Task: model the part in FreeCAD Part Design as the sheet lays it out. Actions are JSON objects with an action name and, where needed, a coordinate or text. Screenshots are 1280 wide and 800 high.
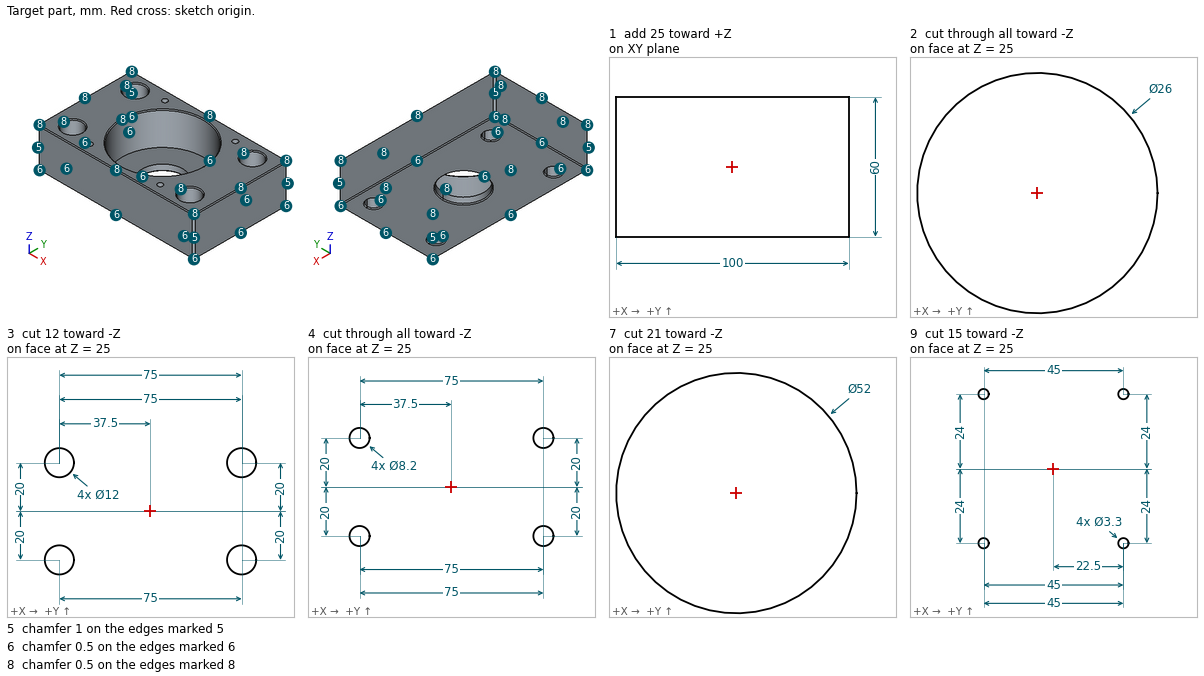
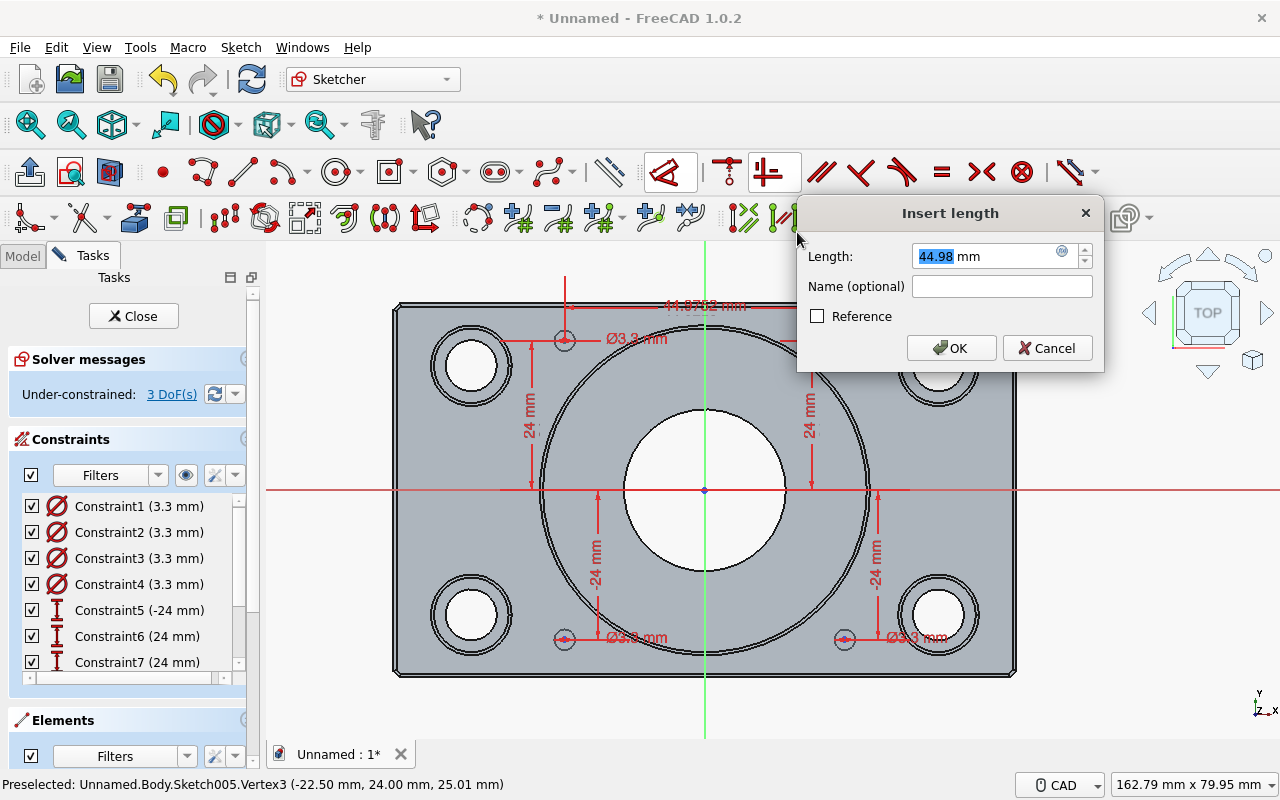
{"action": "type", "text": "45"}
{"action": "key", "text": "Return"}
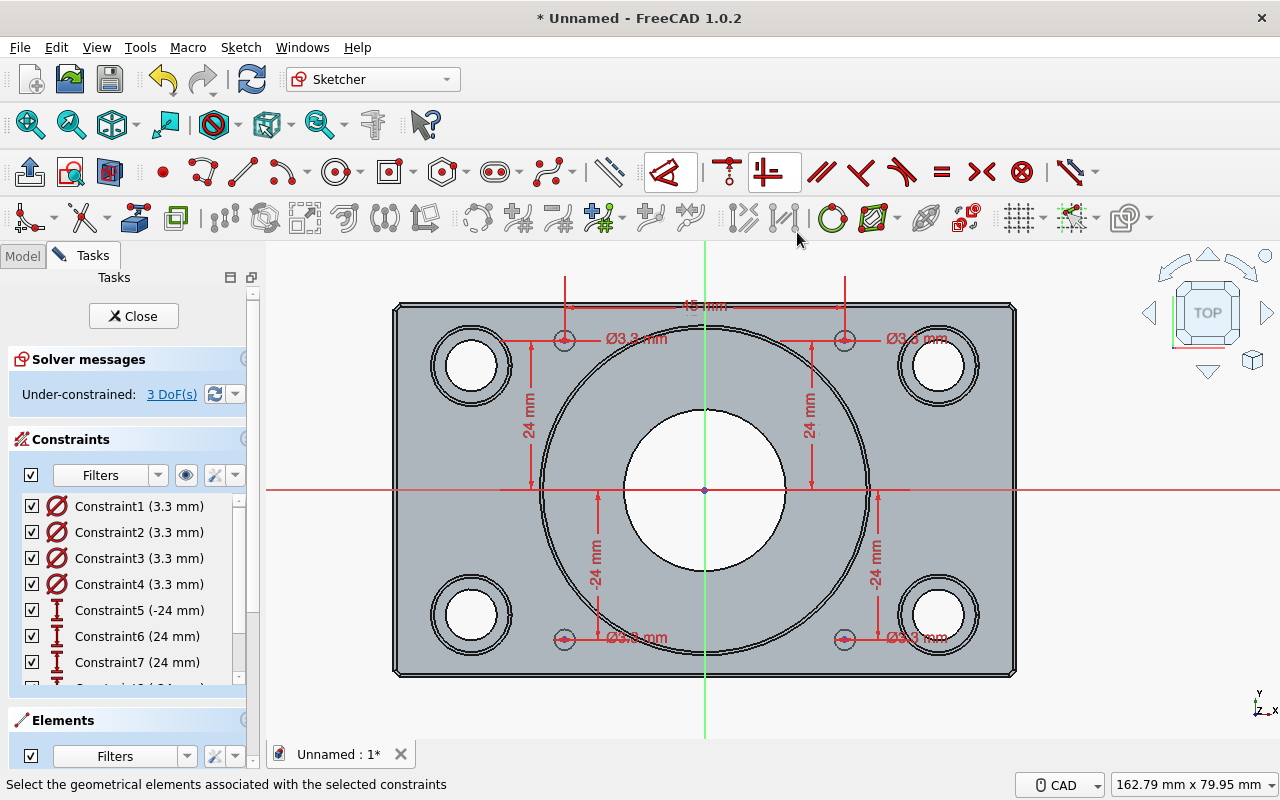
{"action": "left_click", "coordinate": [845, 640]}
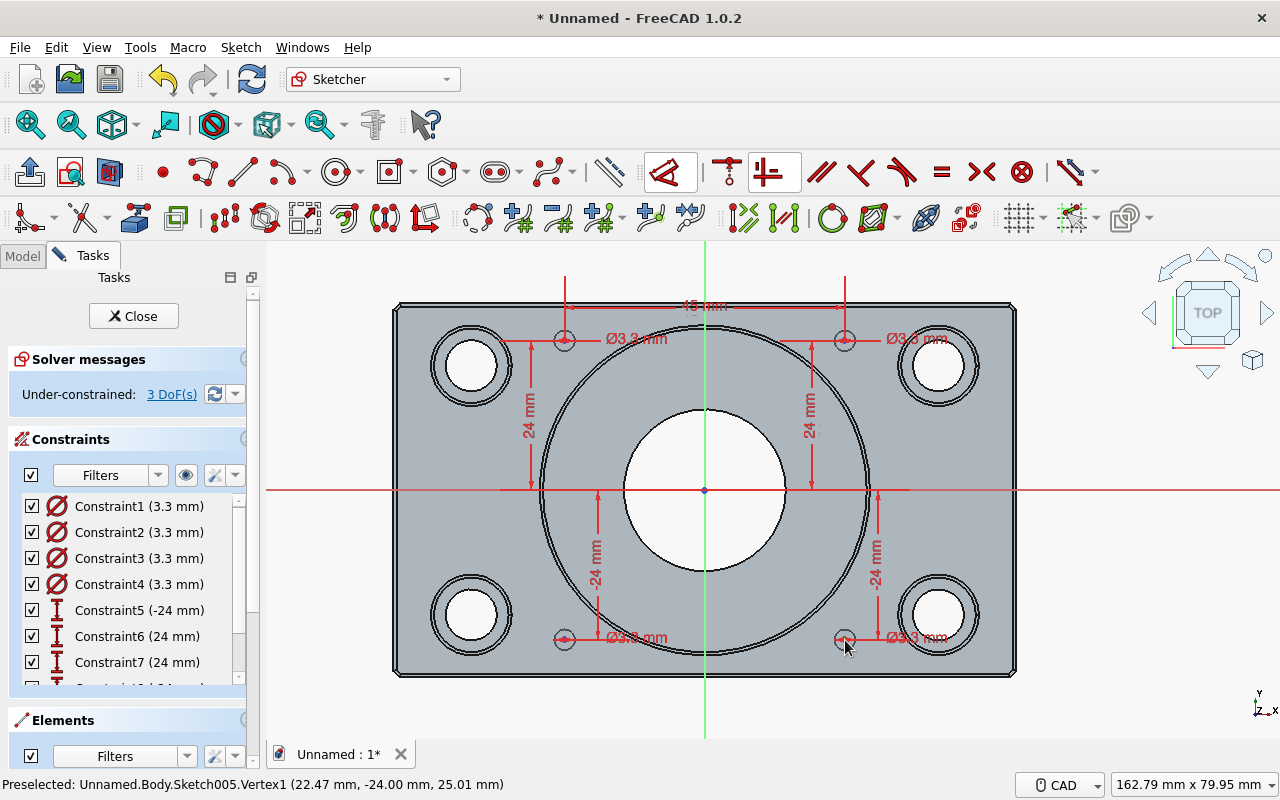
{"action": "left_click", "coordinate": [565, 341]}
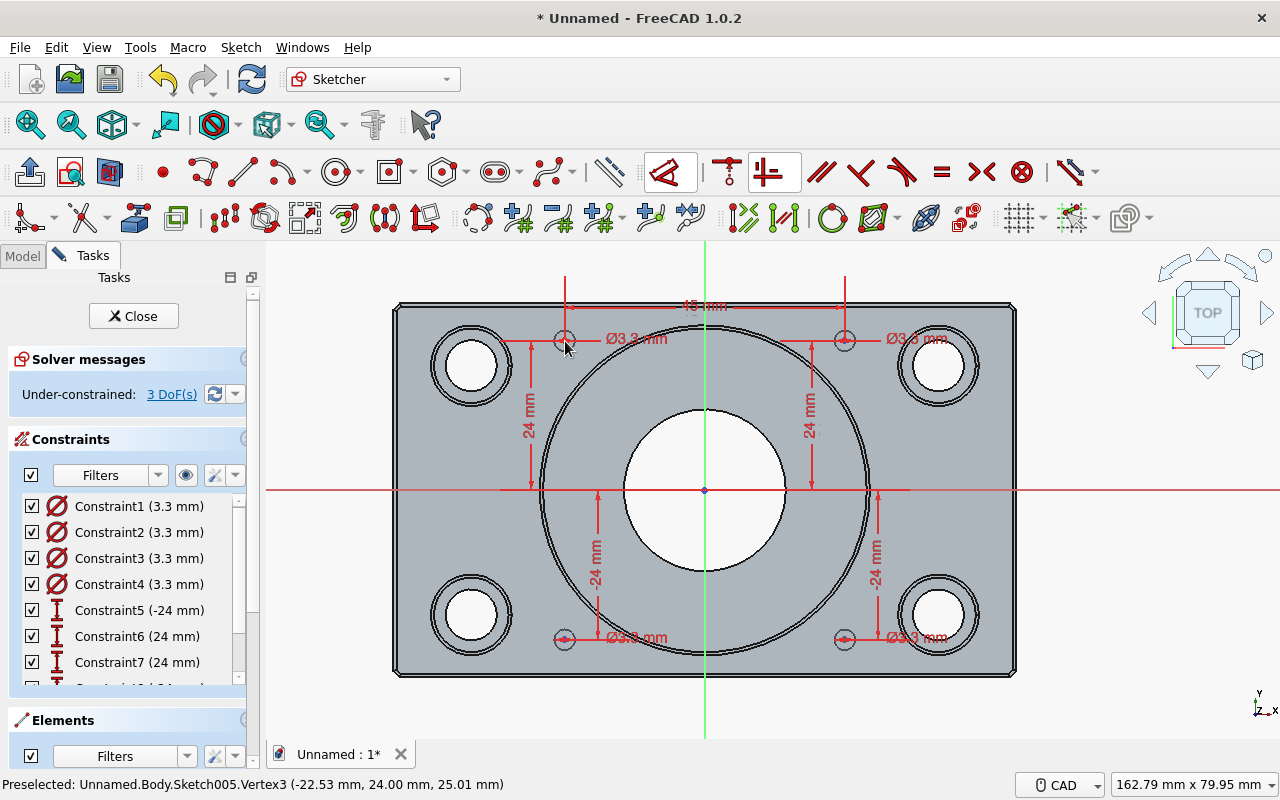
{"action": "left_click", "coordinate": [692, 172]}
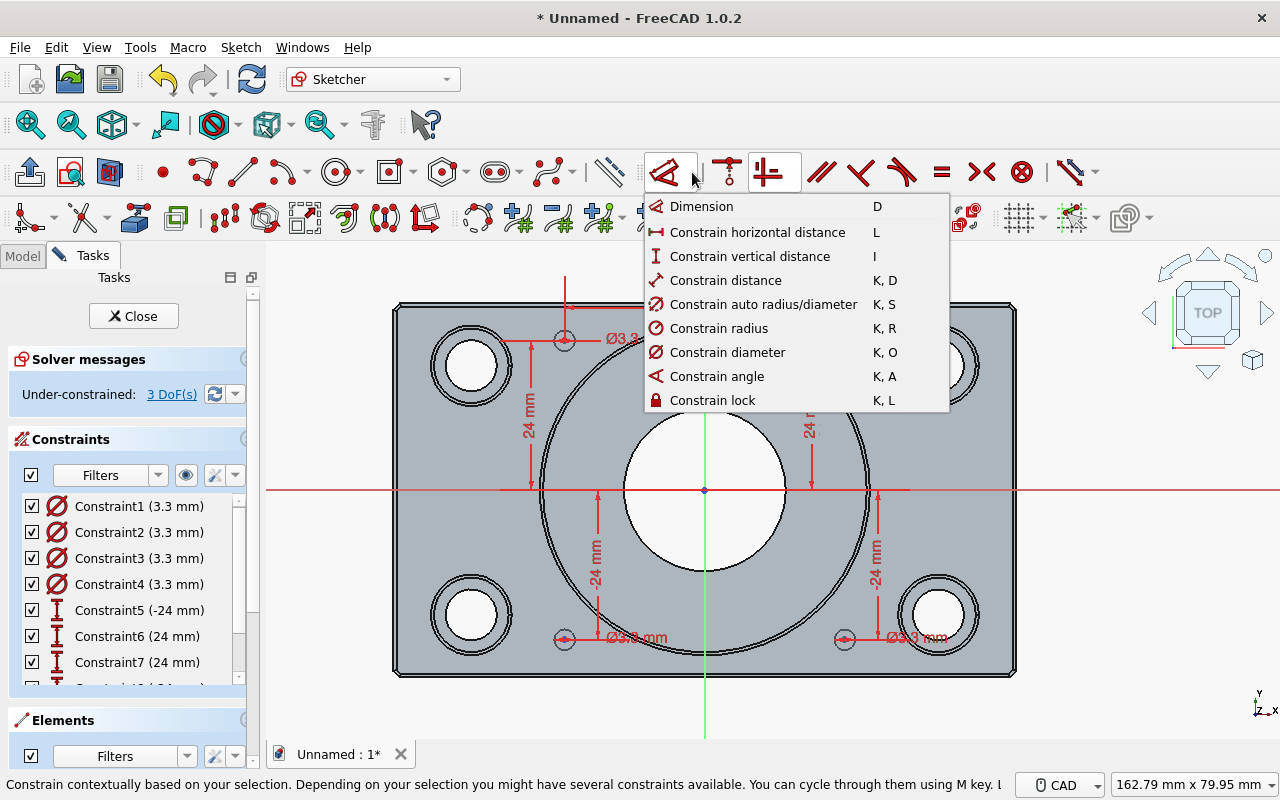
{"action": "left_click", "coordinate": [797, 232]}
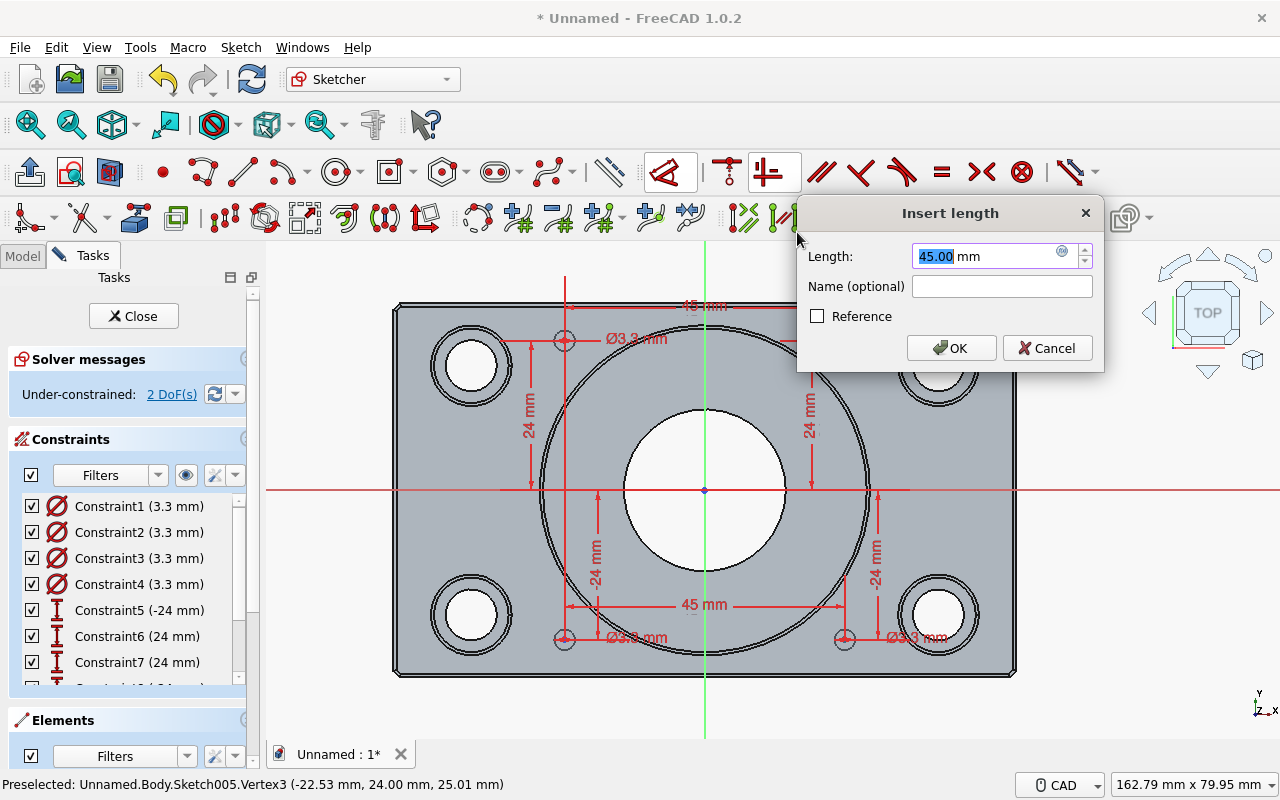
{"action": "type", "text": "45"}
{"action": "key", "text": "Return"}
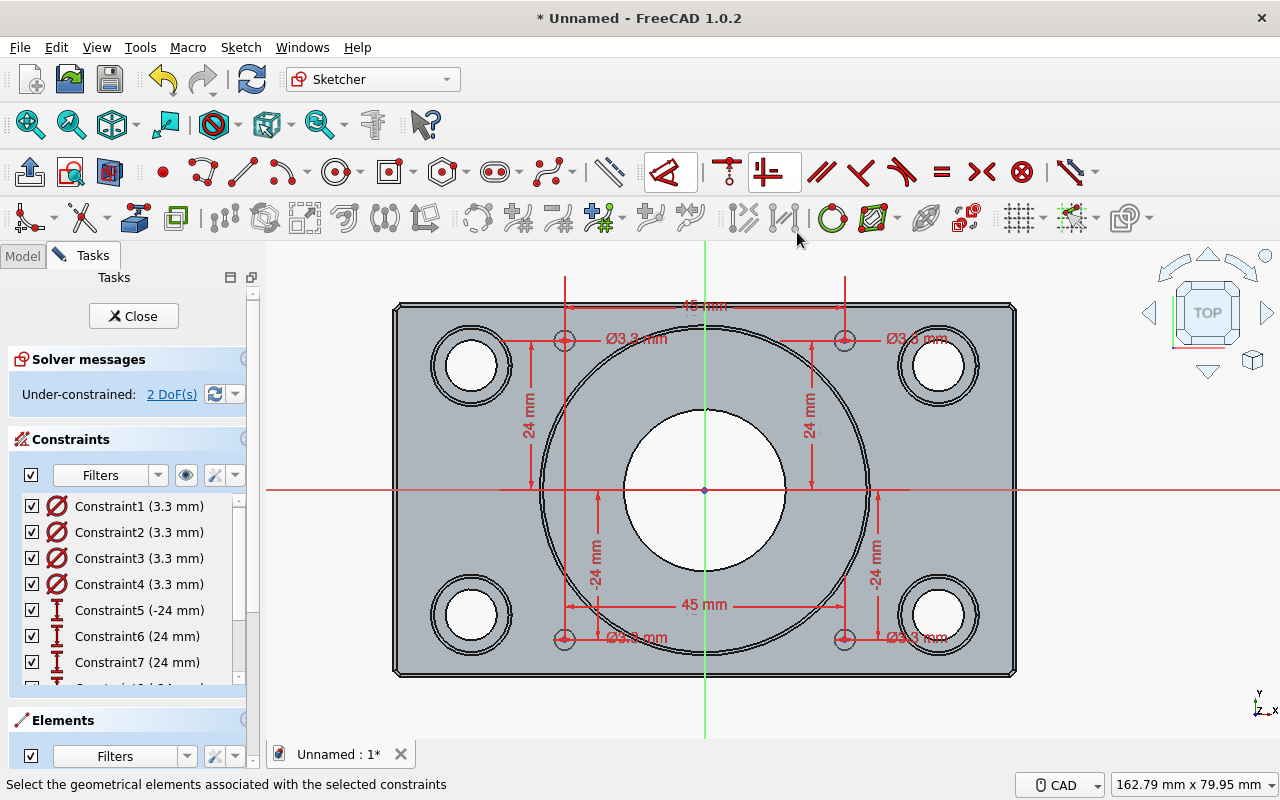
{"action": "left_click", "coordinate": [845, 640]}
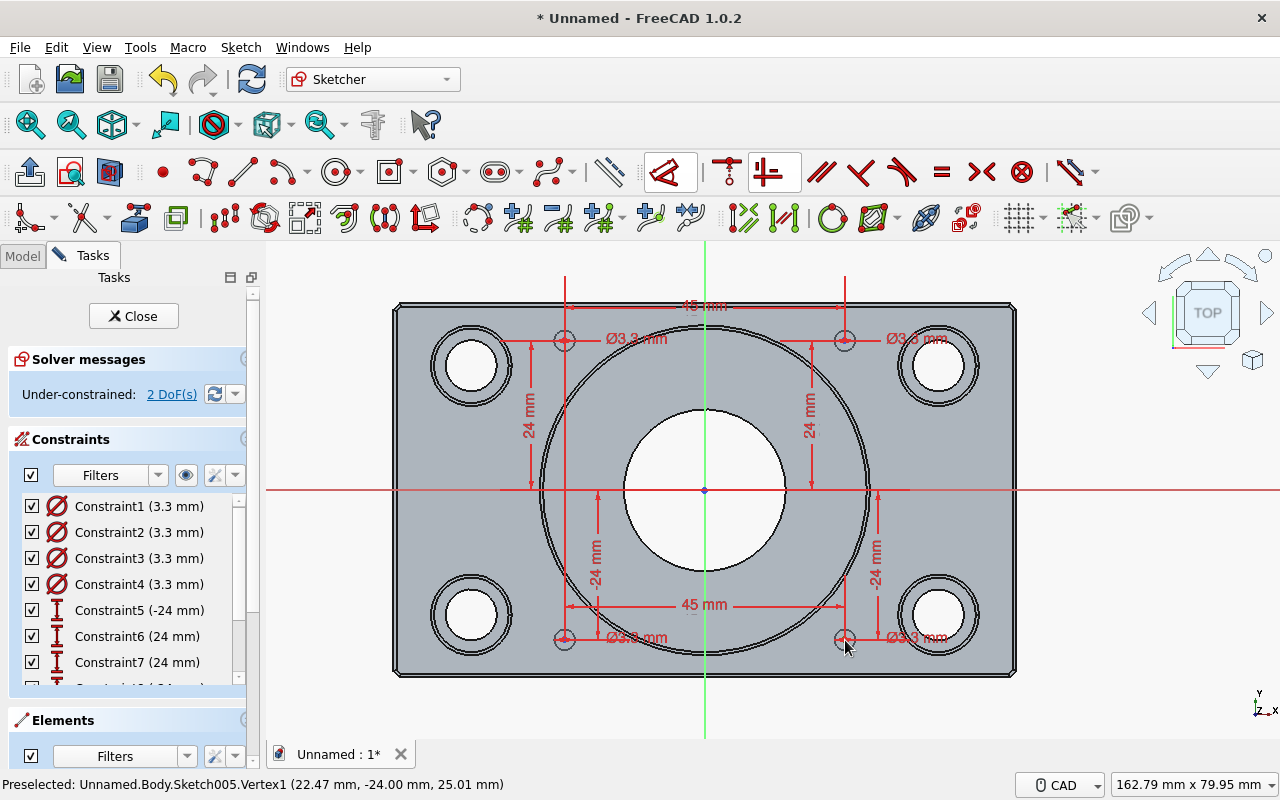
{"action": "left_click", "coordinate": [565, 640]}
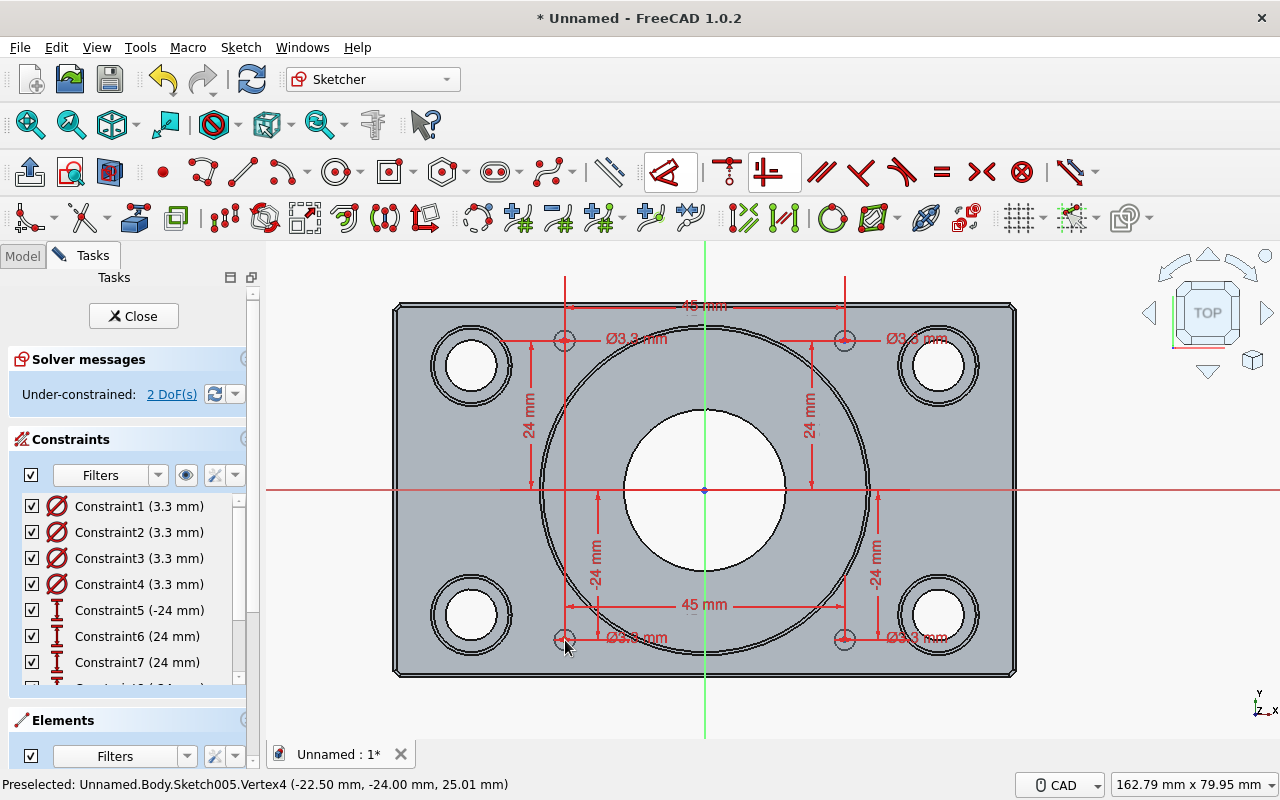
{"action": "key", "text": "l"}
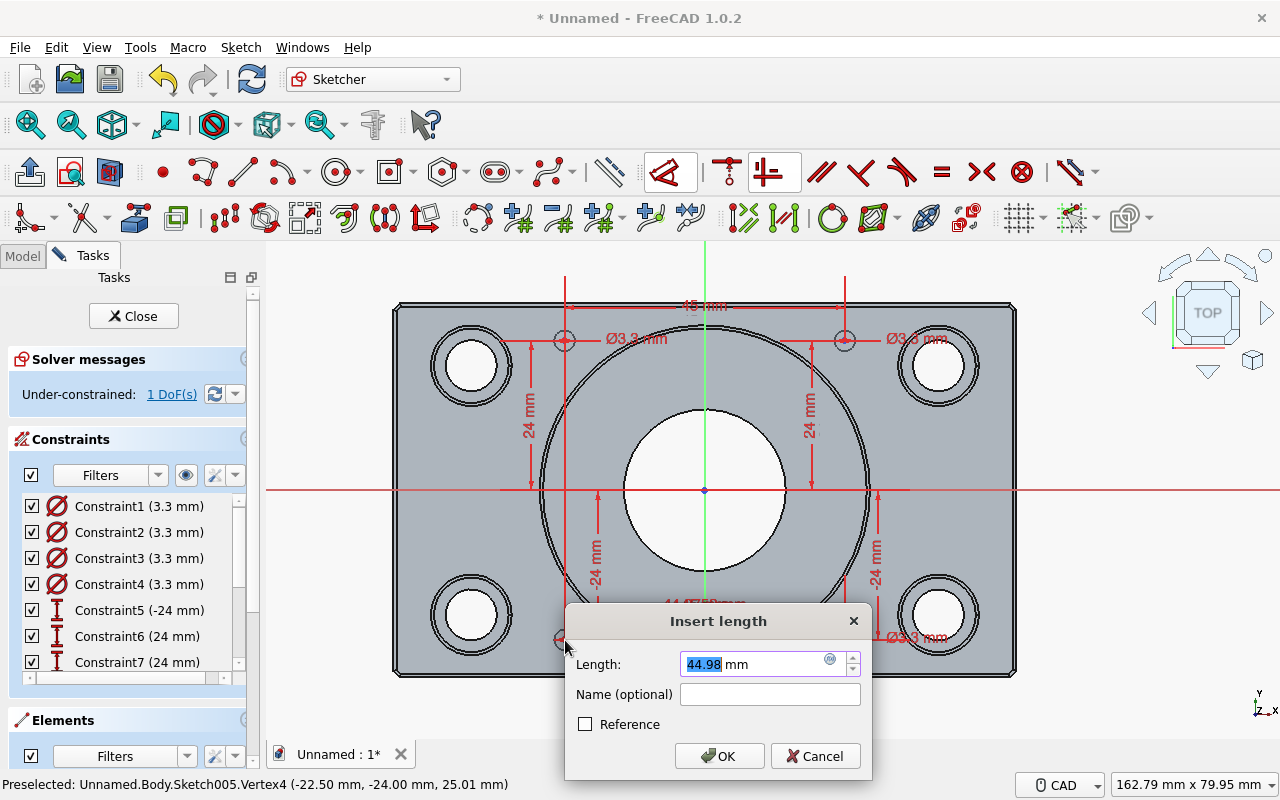
{"action": "type", "text": "45"}
{"action": "key", "text": "Return"}